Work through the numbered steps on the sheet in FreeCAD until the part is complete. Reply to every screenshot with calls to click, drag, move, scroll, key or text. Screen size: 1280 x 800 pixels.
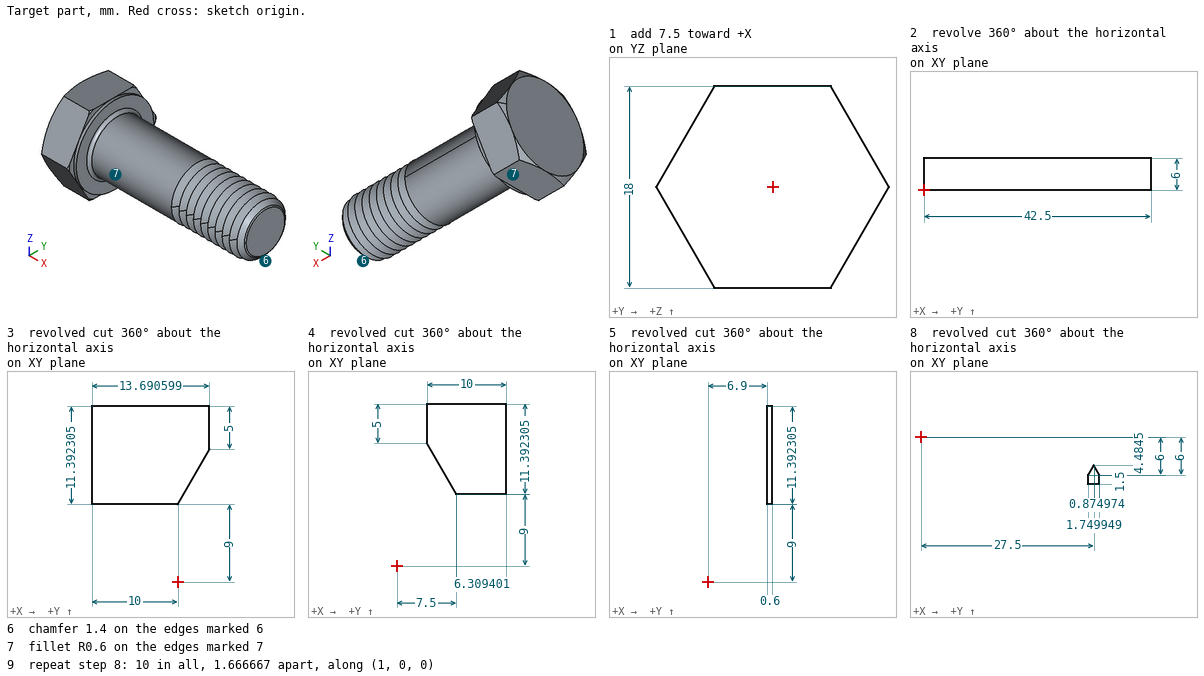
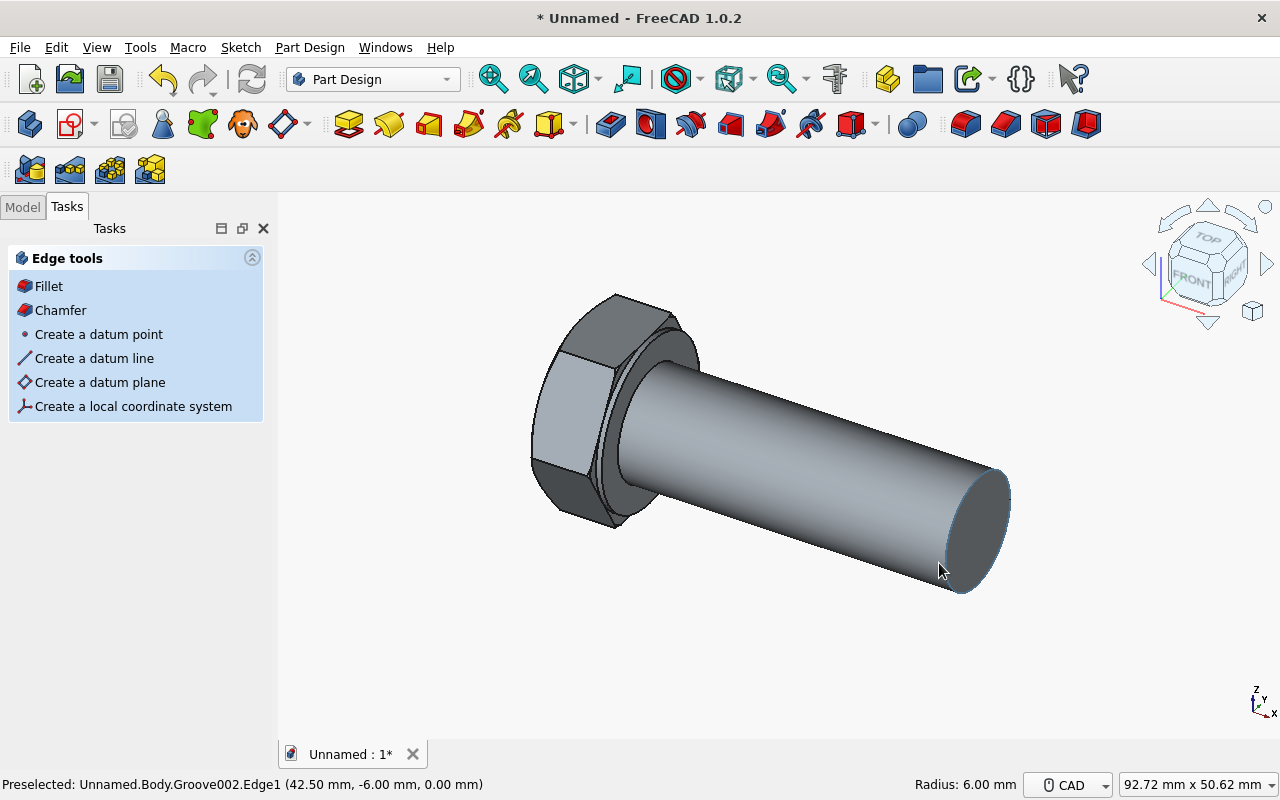
click(1006, 124)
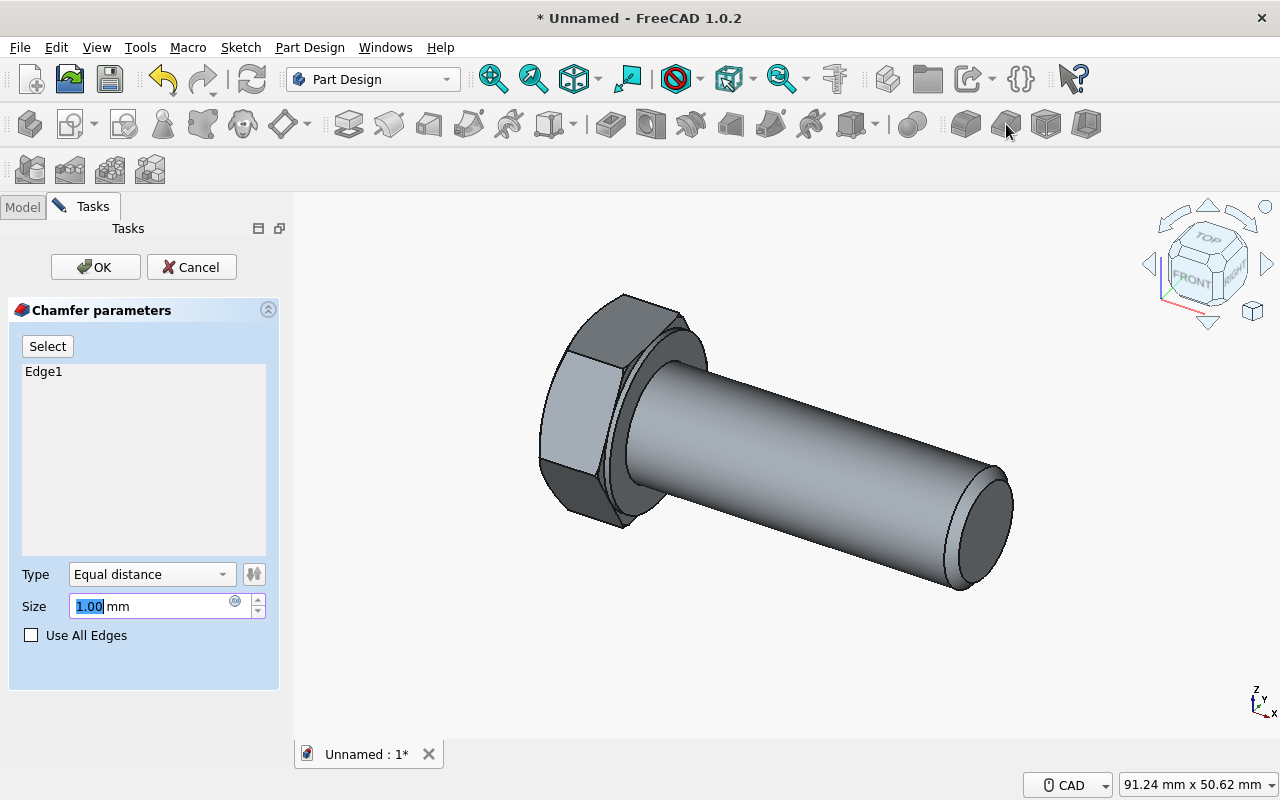
text(1.4)
key(Tab)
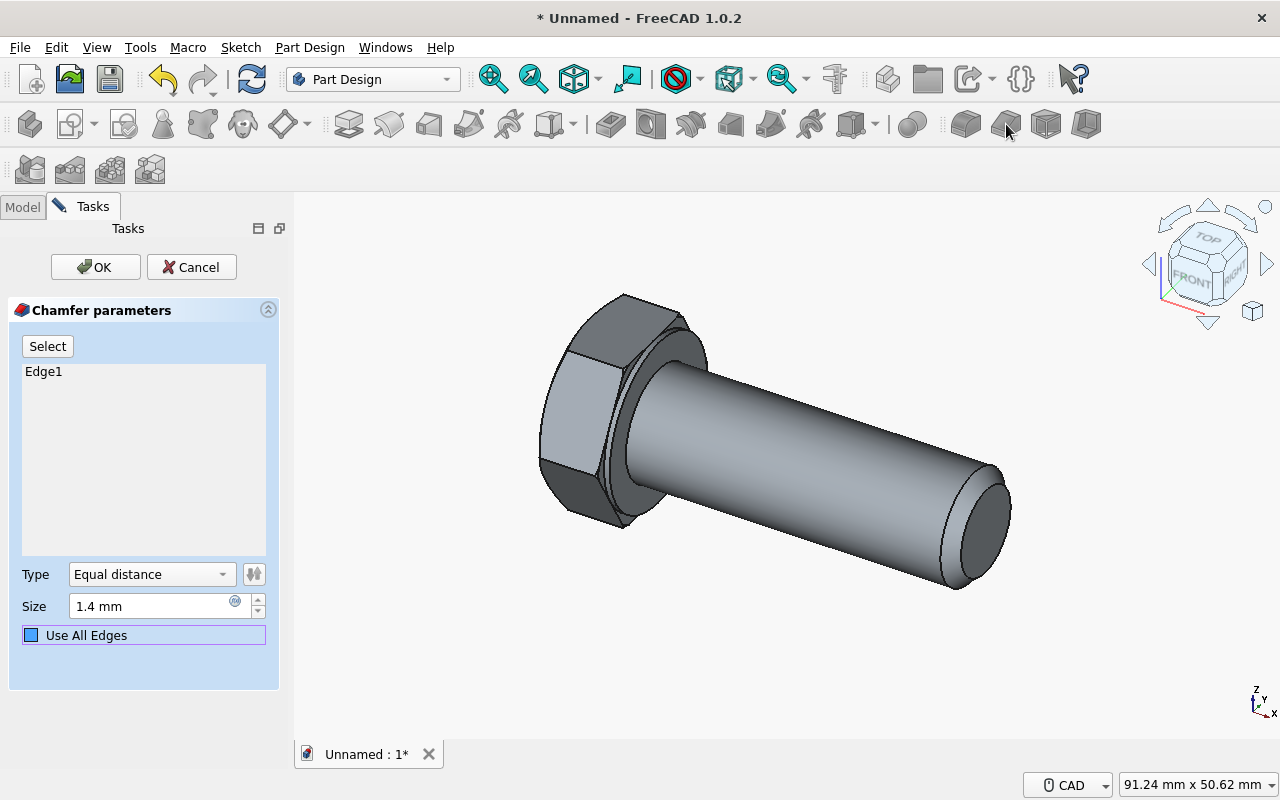
click(96, 267)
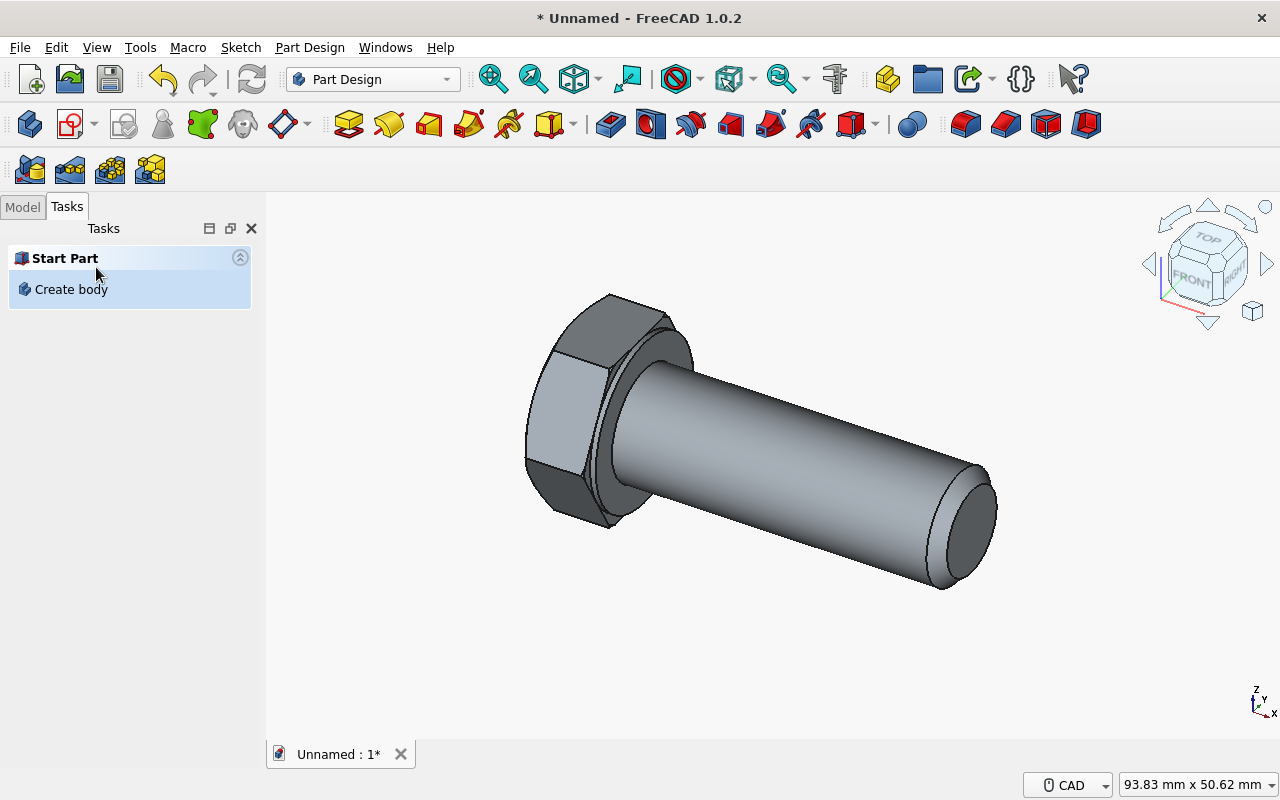
key(0)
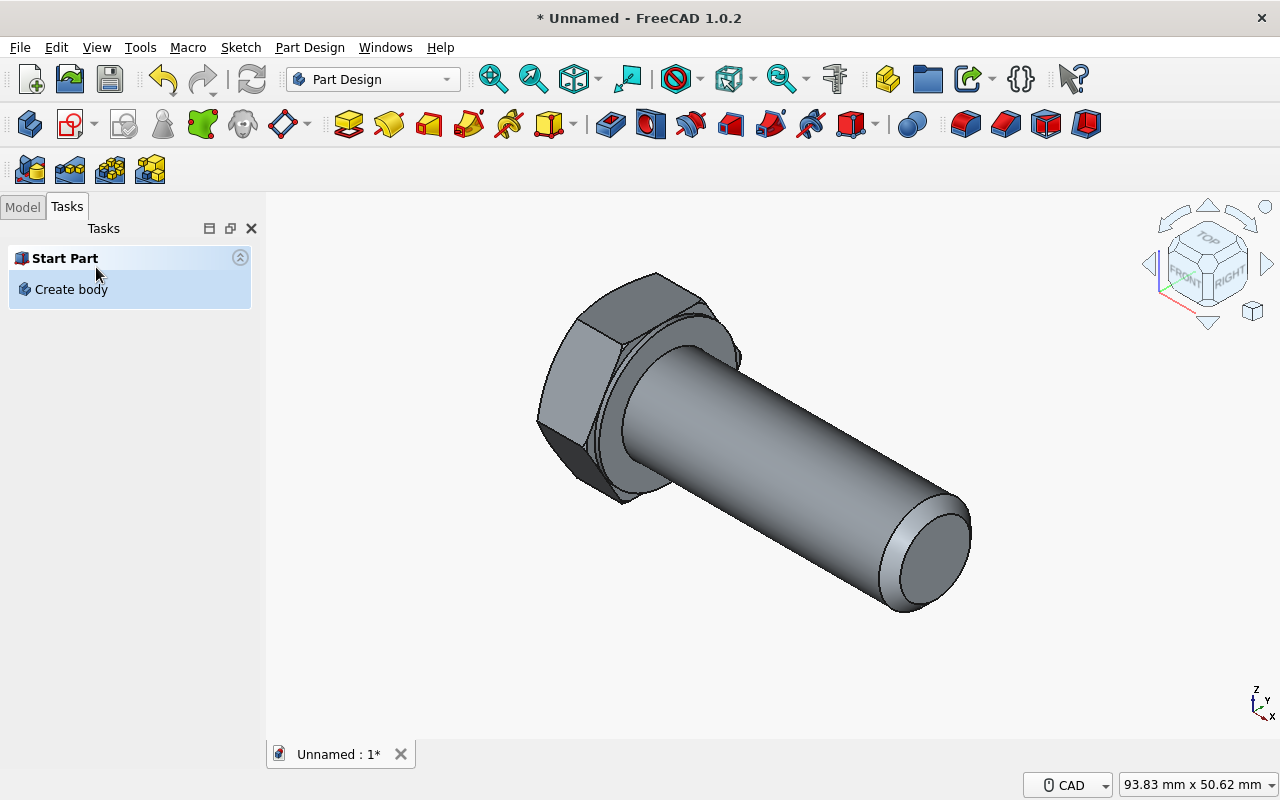
key(2)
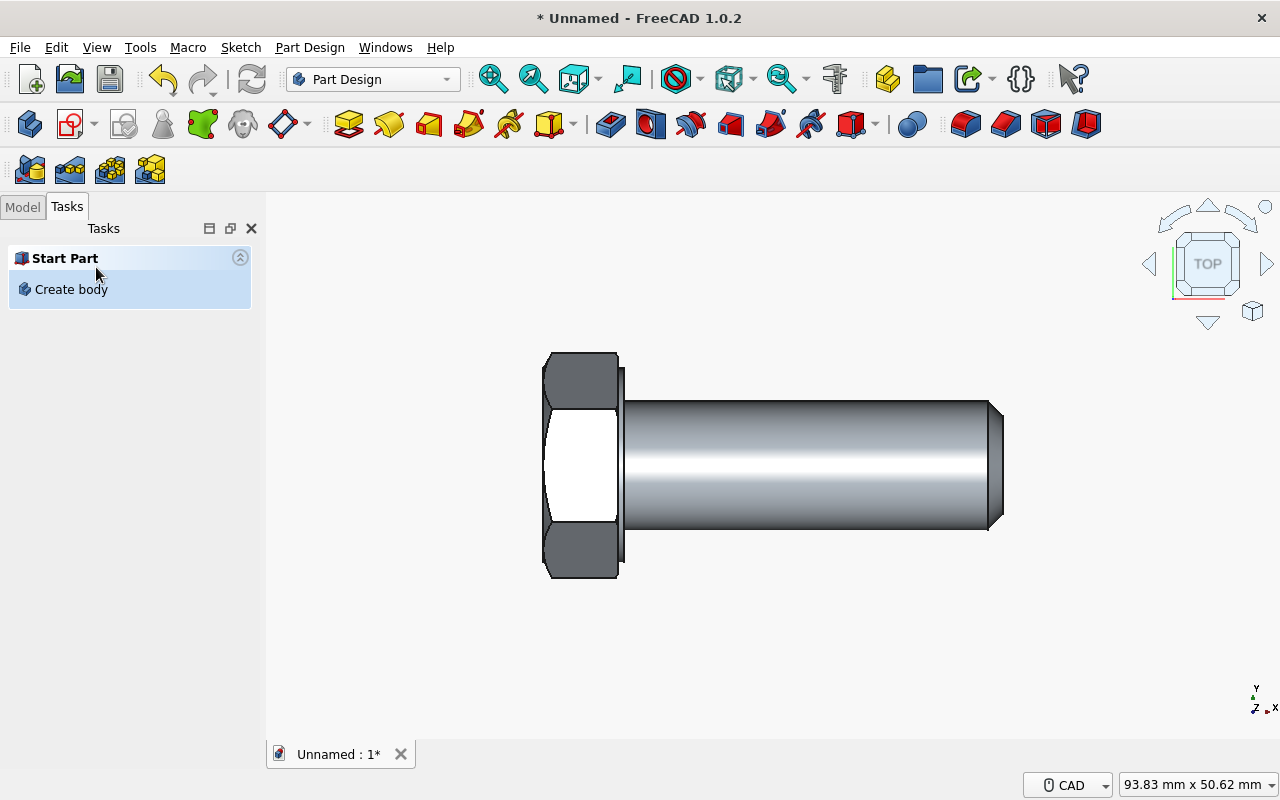
key(1)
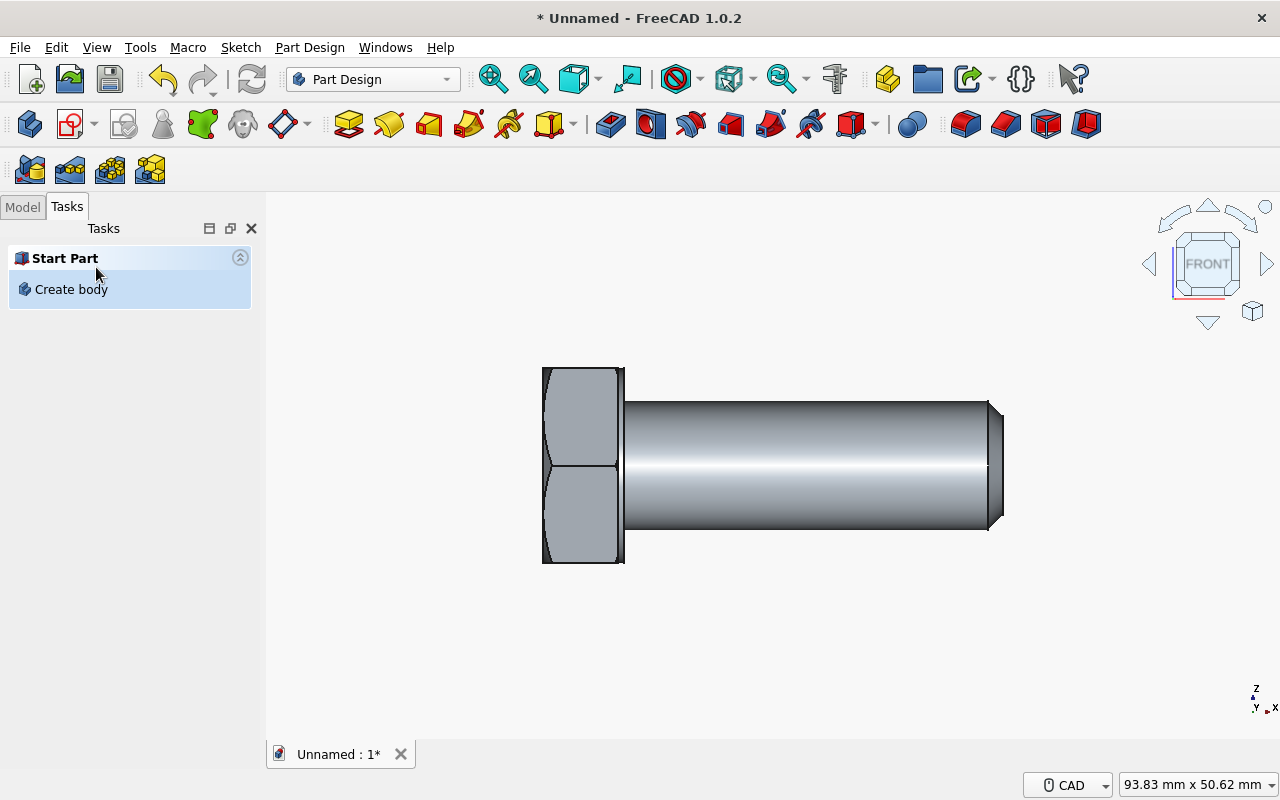
key(3)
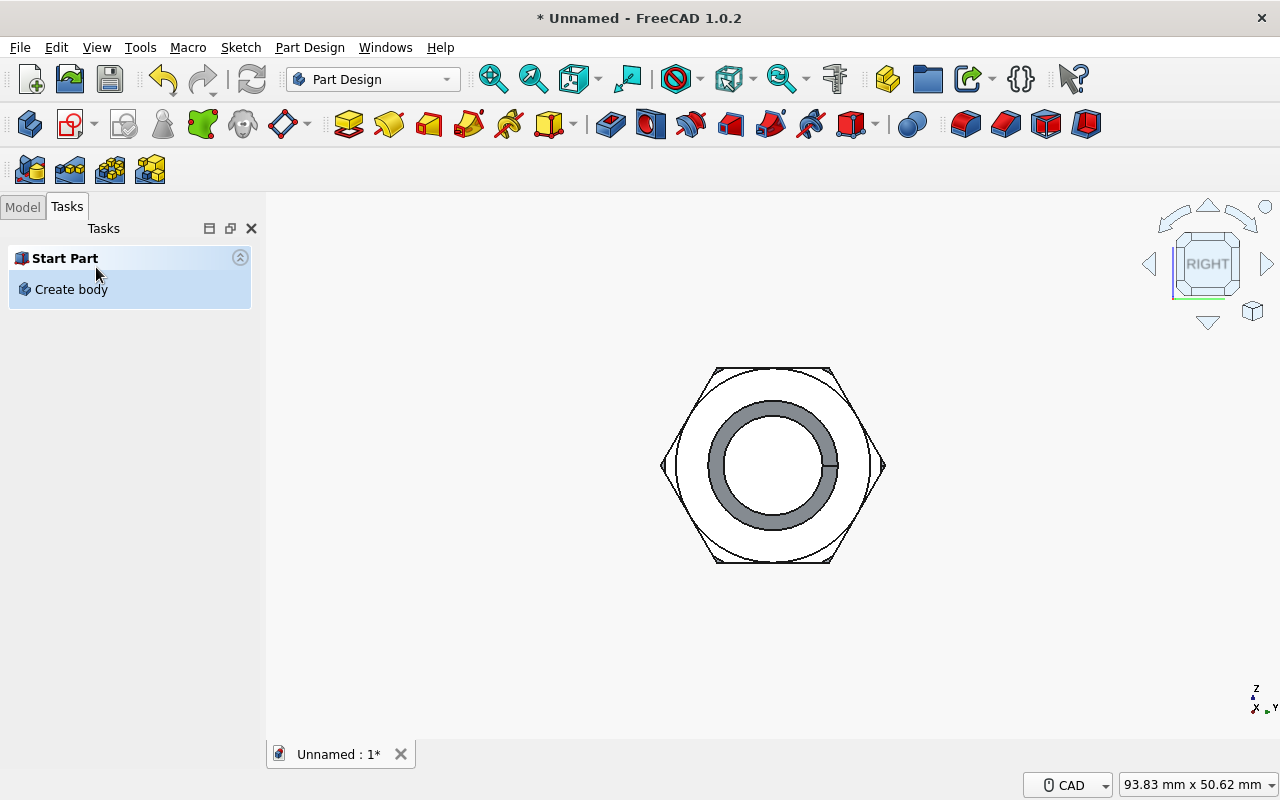
key(v)
key(f)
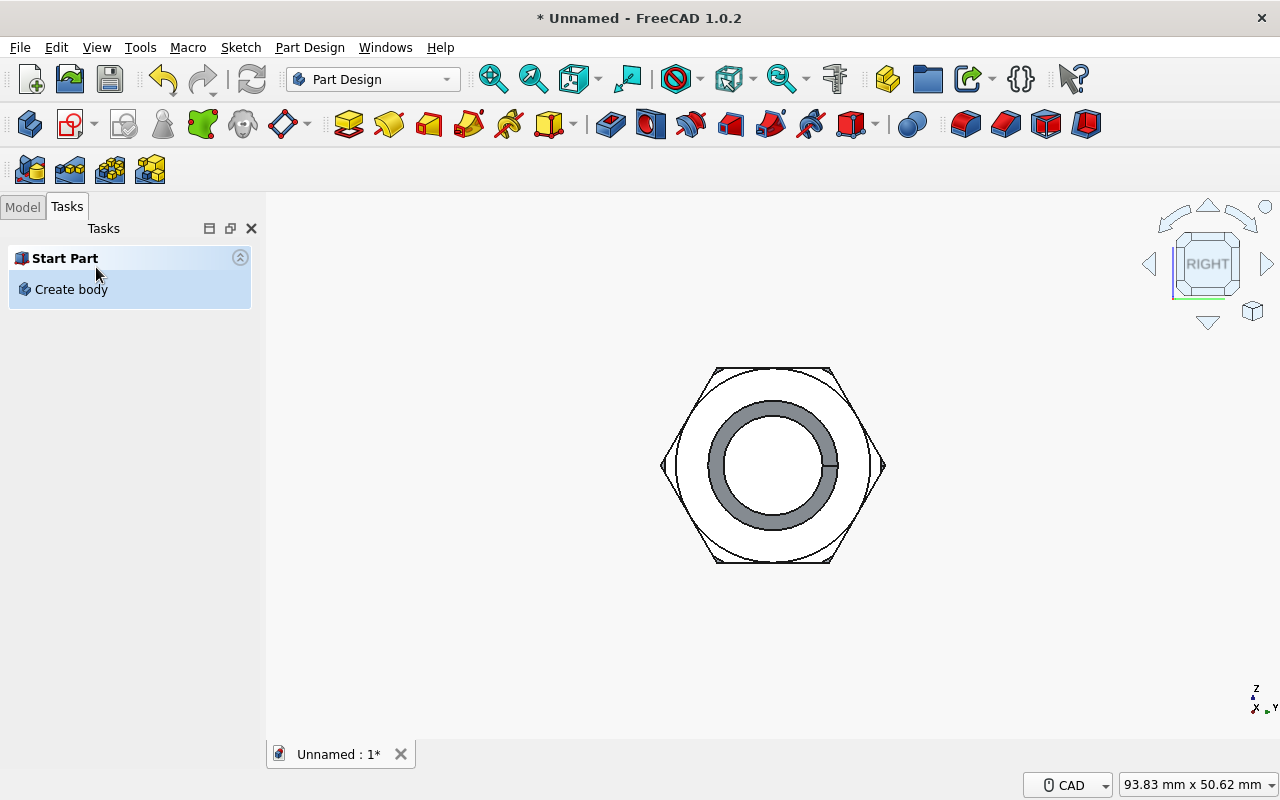
key(5)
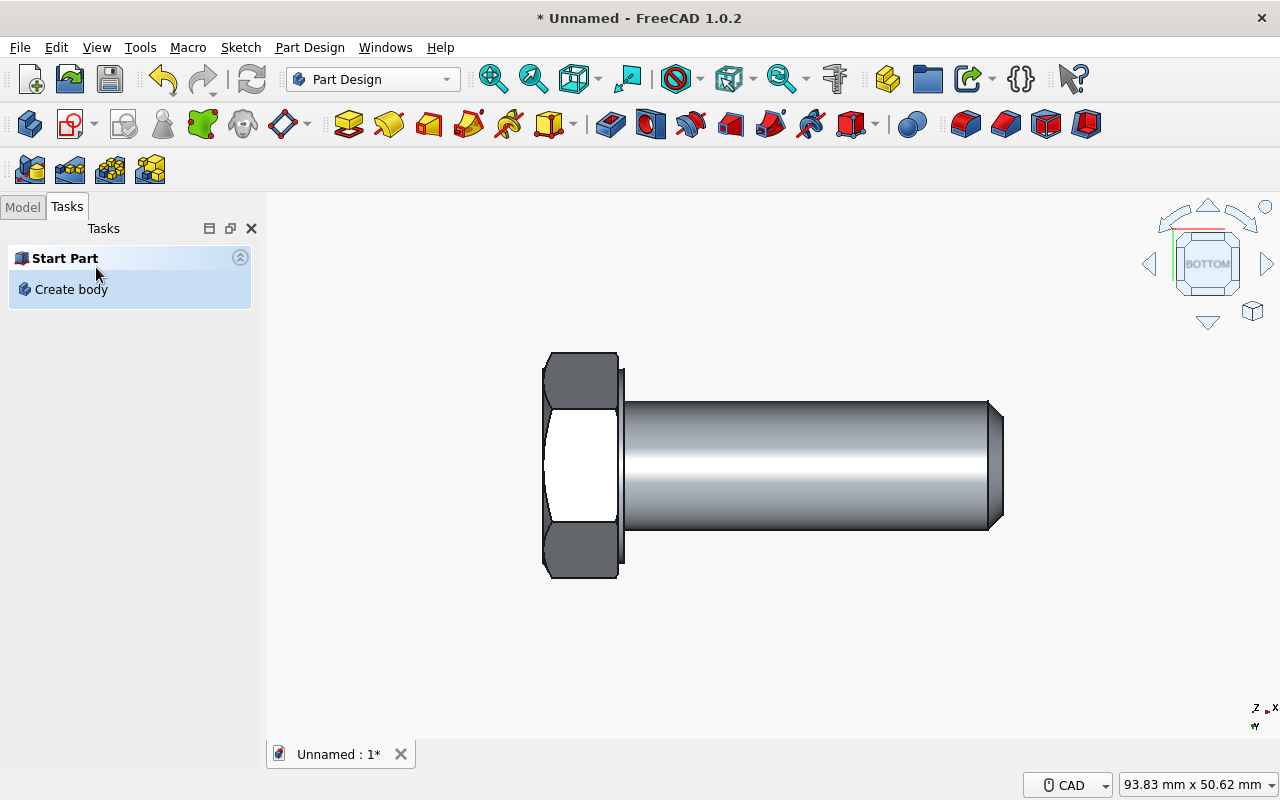
key(4)